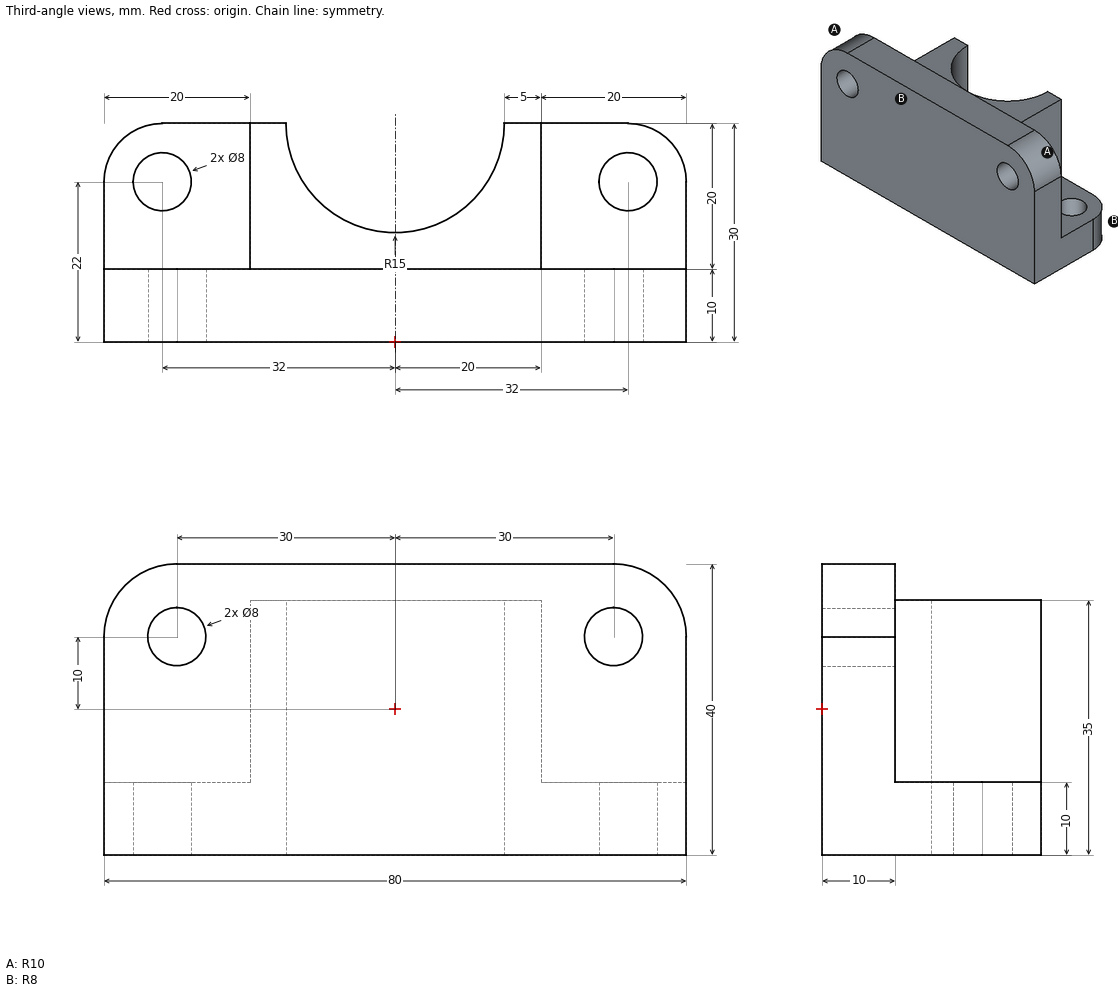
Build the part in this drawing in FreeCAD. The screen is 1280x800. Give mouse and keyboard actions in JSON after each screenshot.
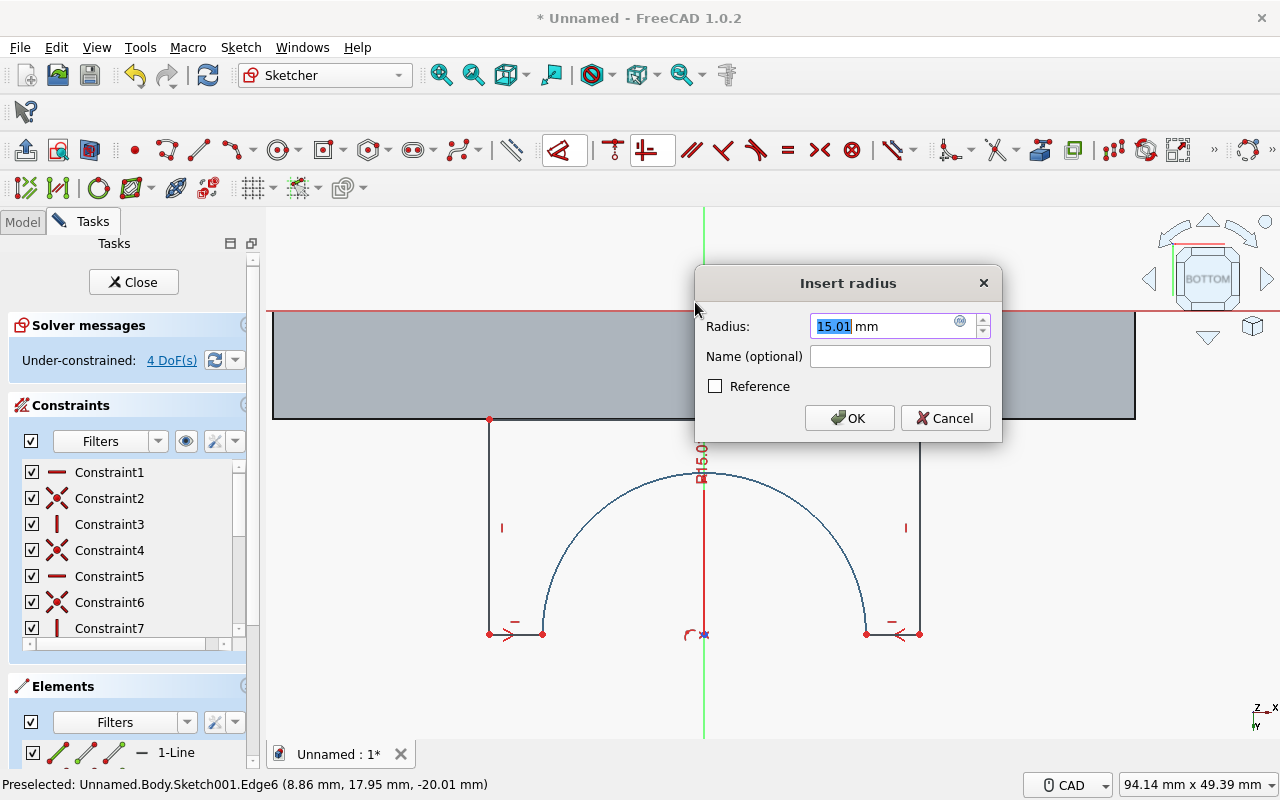
{"action": "type", "text": "15"}
{"action": "key", "text": "Return"}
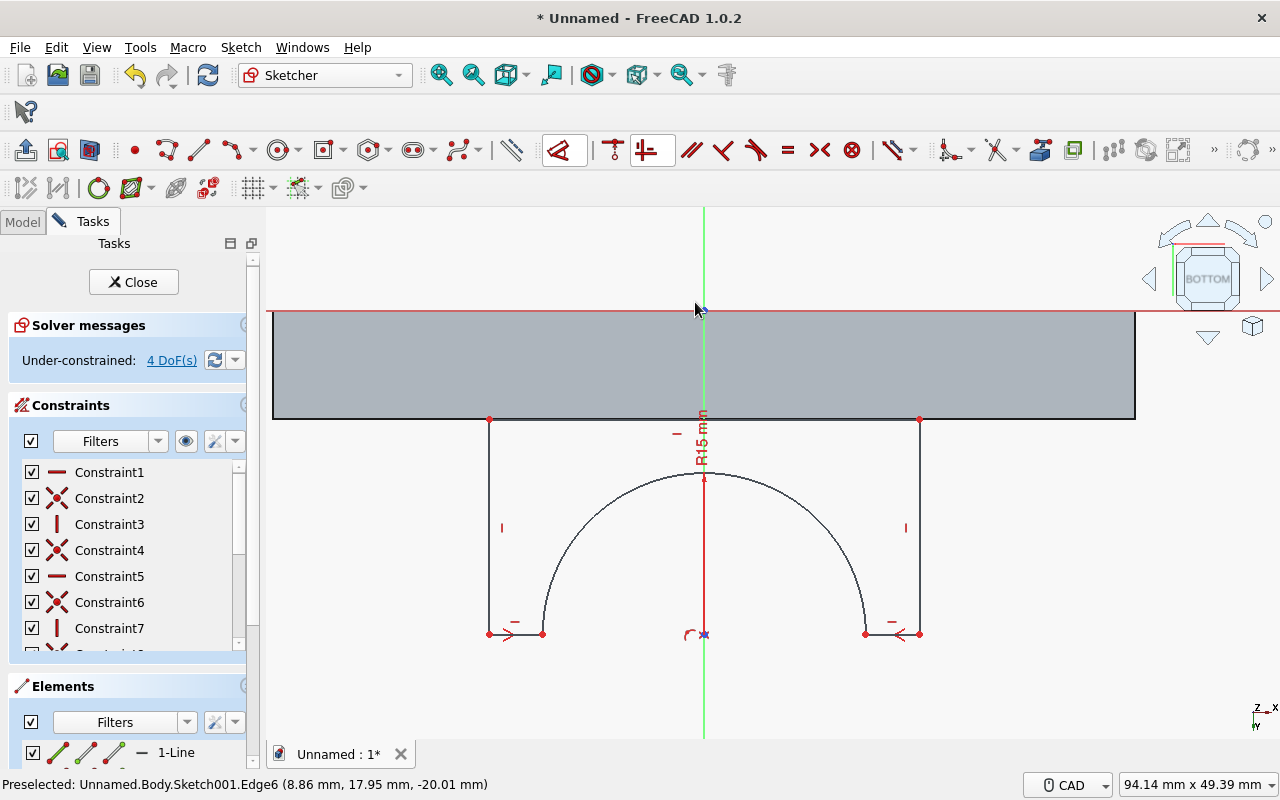
{"action": "left_click", "coordinate": [882, 635]}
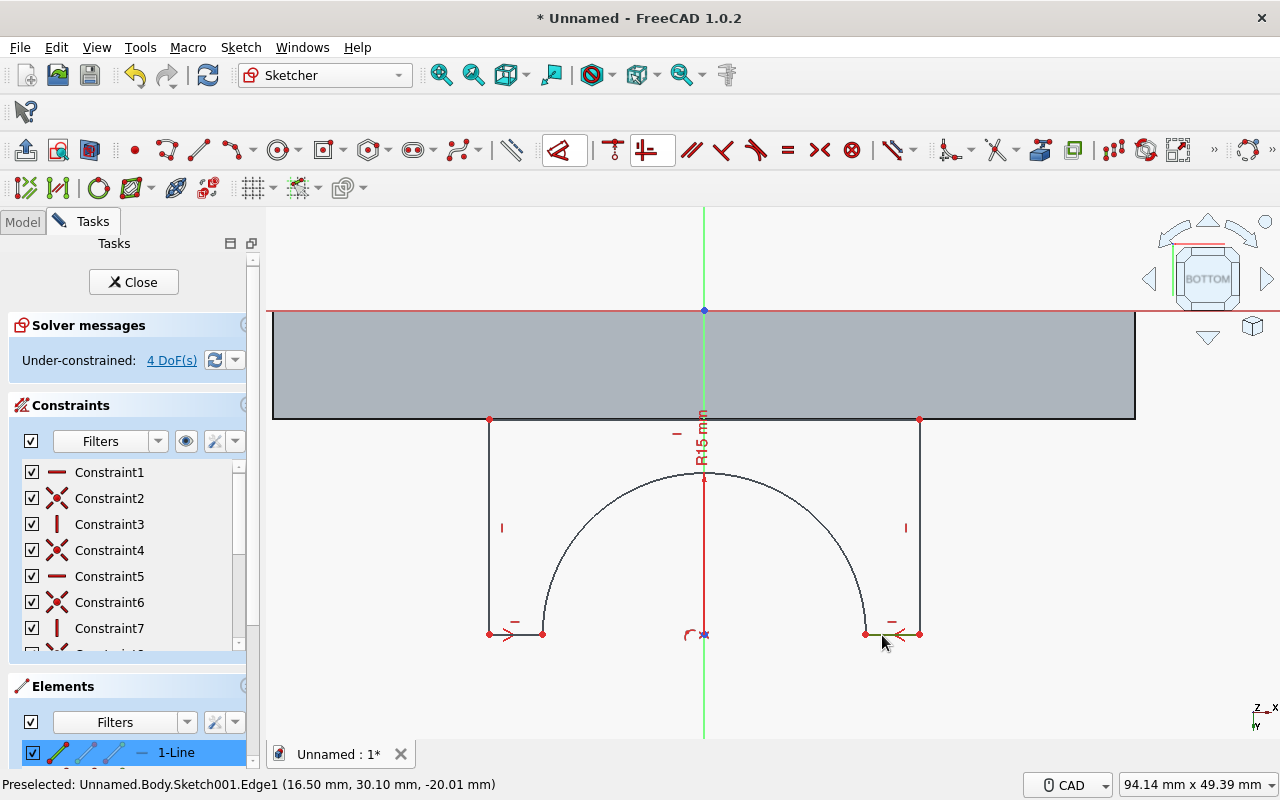
{"action": "left_click", "coordinate": [582, 150]}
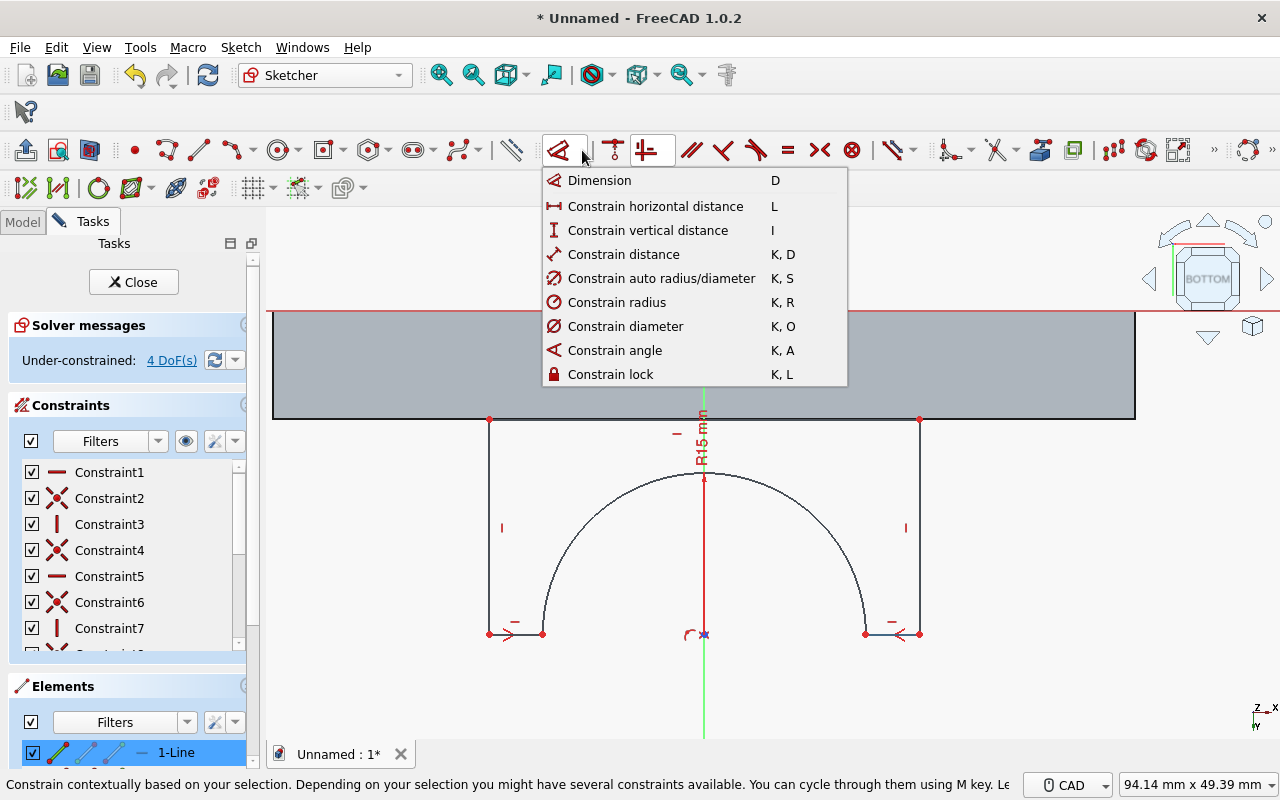
{"action": "left_click", "coordinate": [695, 206]}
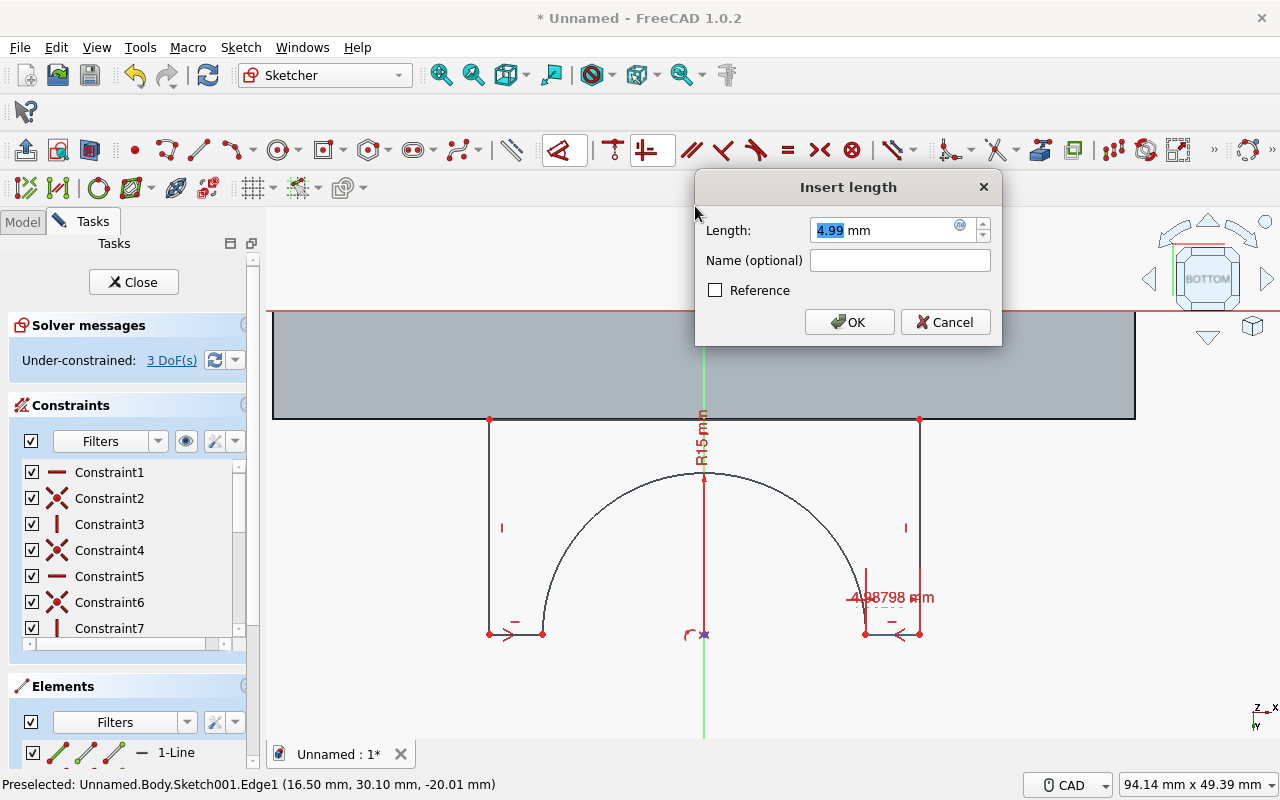
{"action": "type", "text": "5"}
{"action": "key", "text": "Return"}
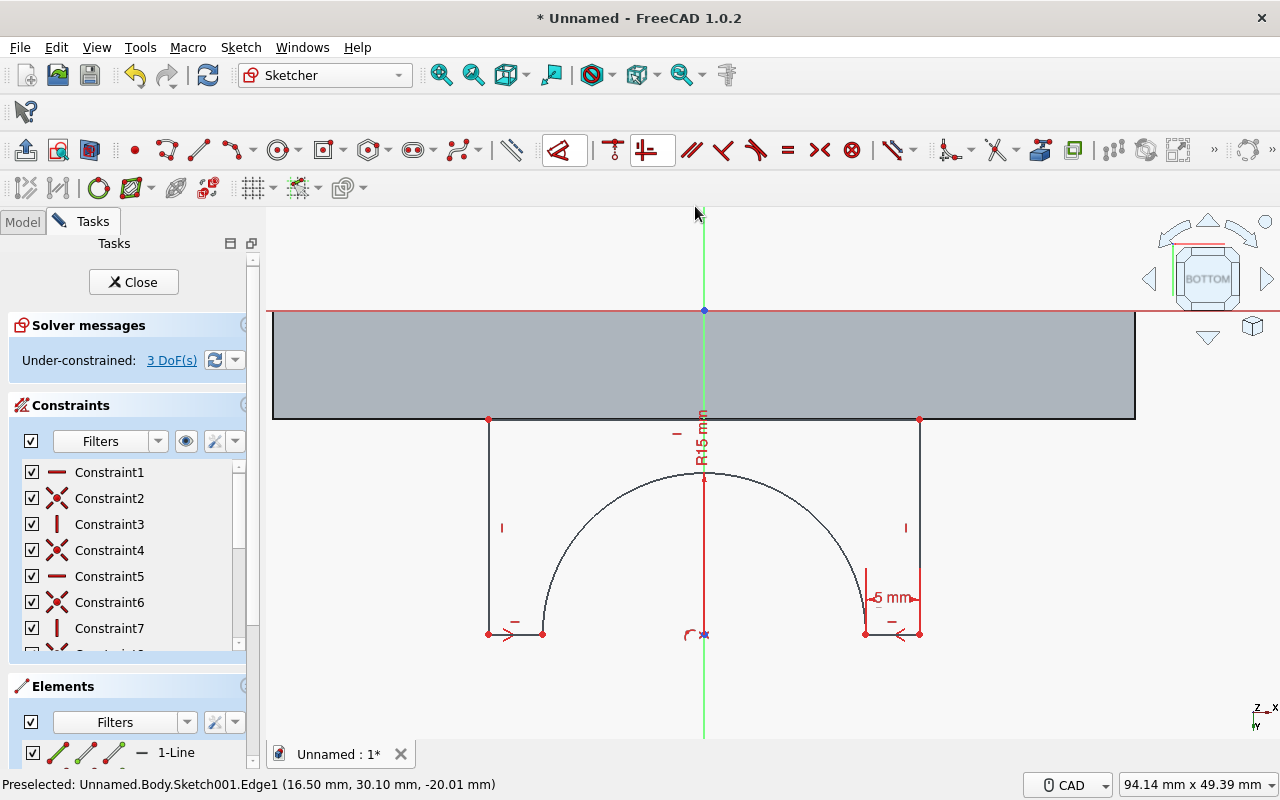
{"action": "left_click", "coordinate": [920, 570]}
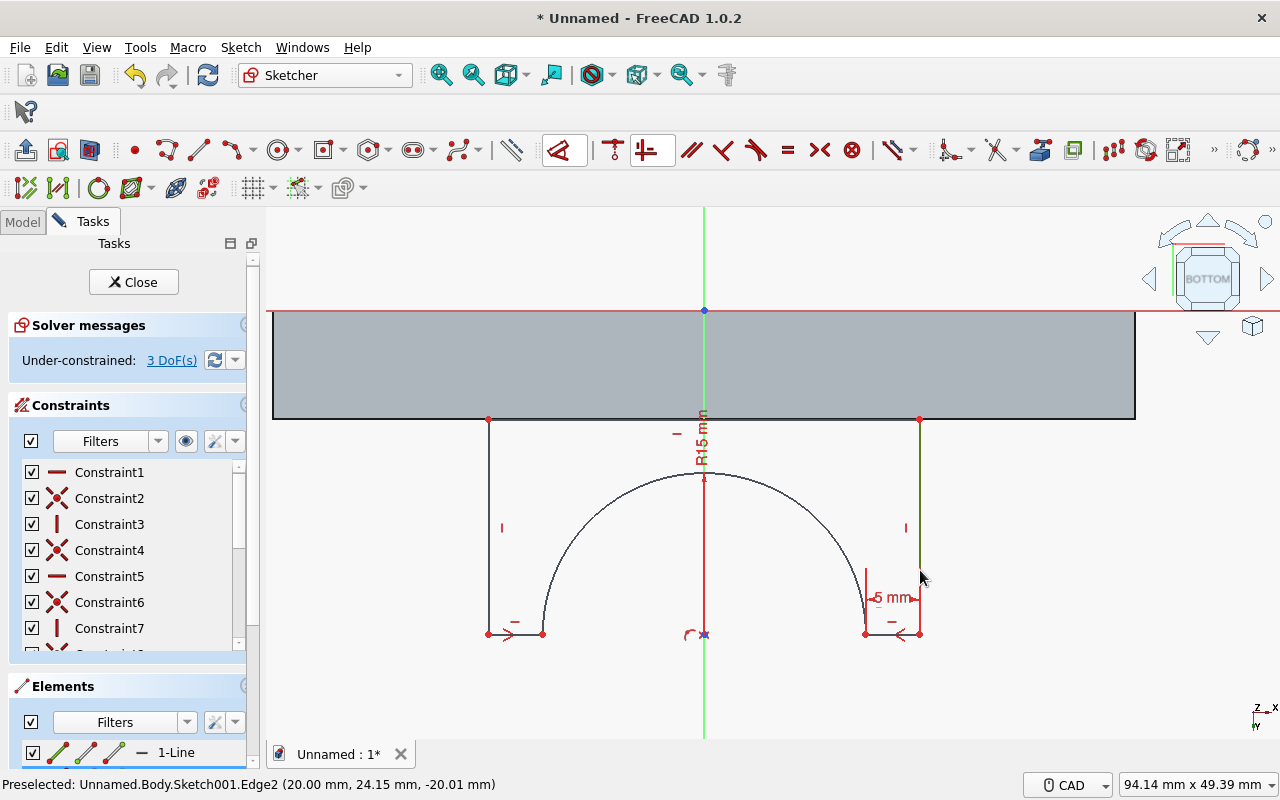
{"action": "left_click", "coordinate": [582, 150]}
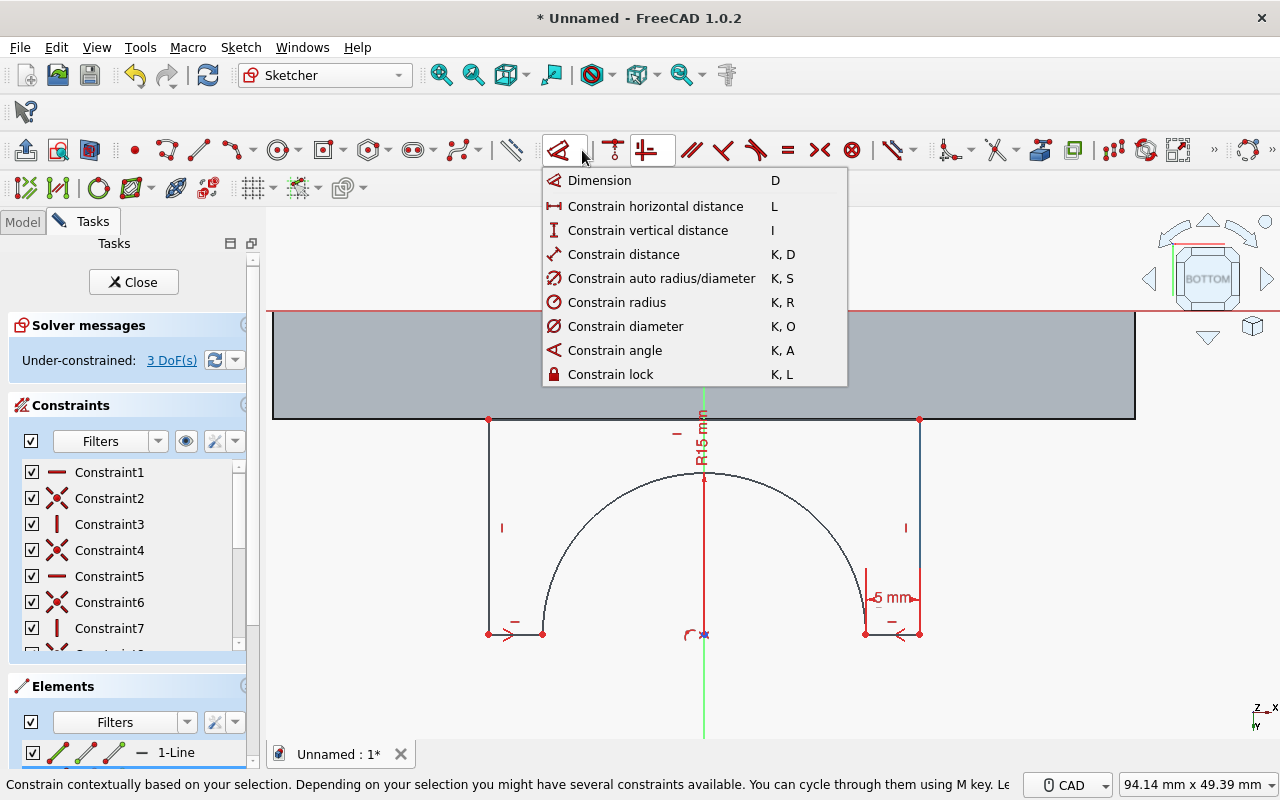
{"action": "left_click", "coordinate": [695, 230]}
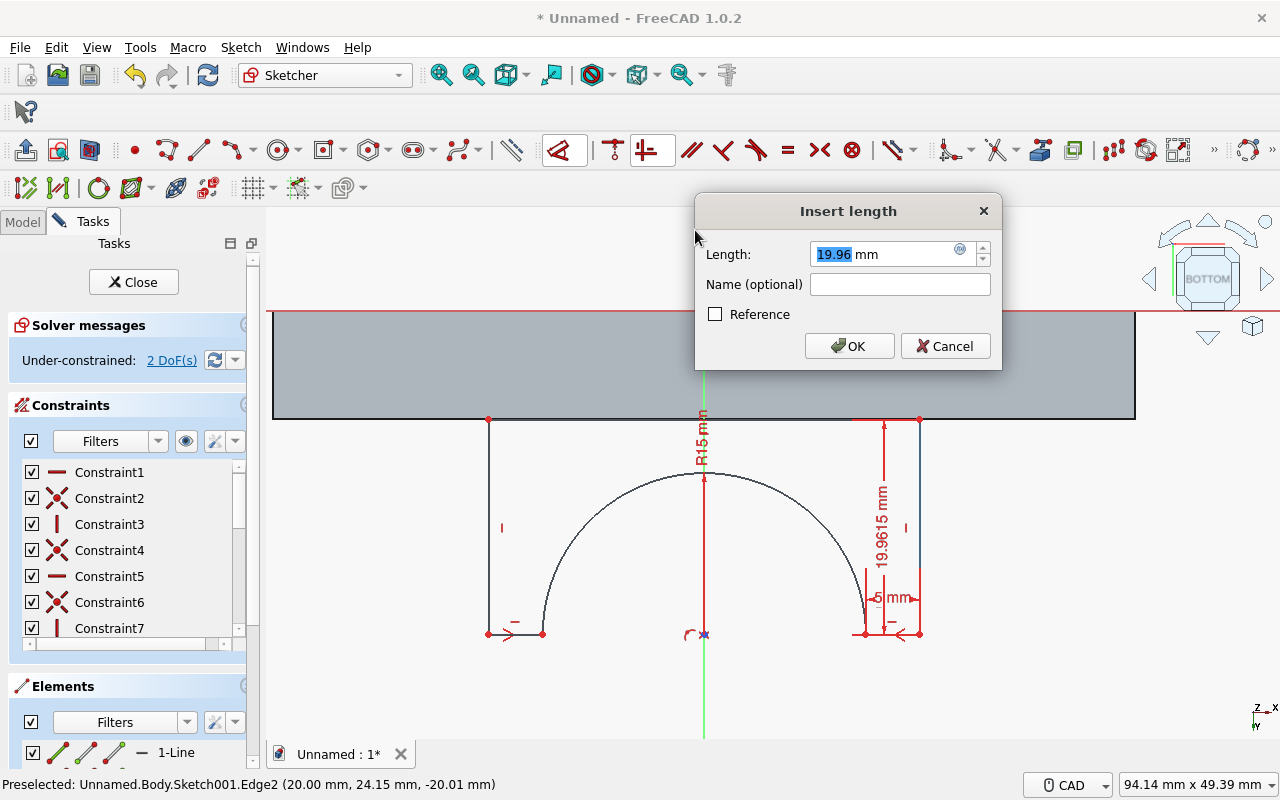
{"action": "type", "text": "20"}
{"action": "key", "text": "Return"}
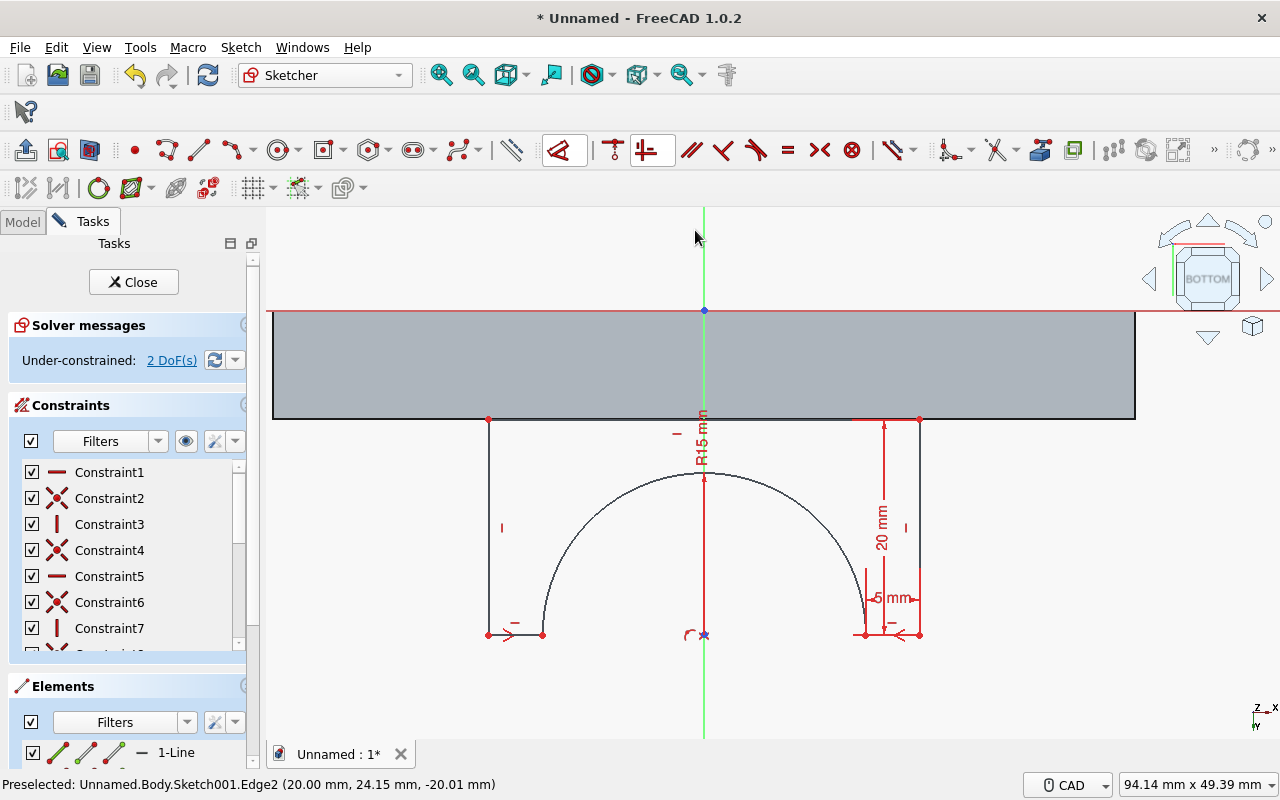
{"action": "left_click", "coordinate": [866, 635]}